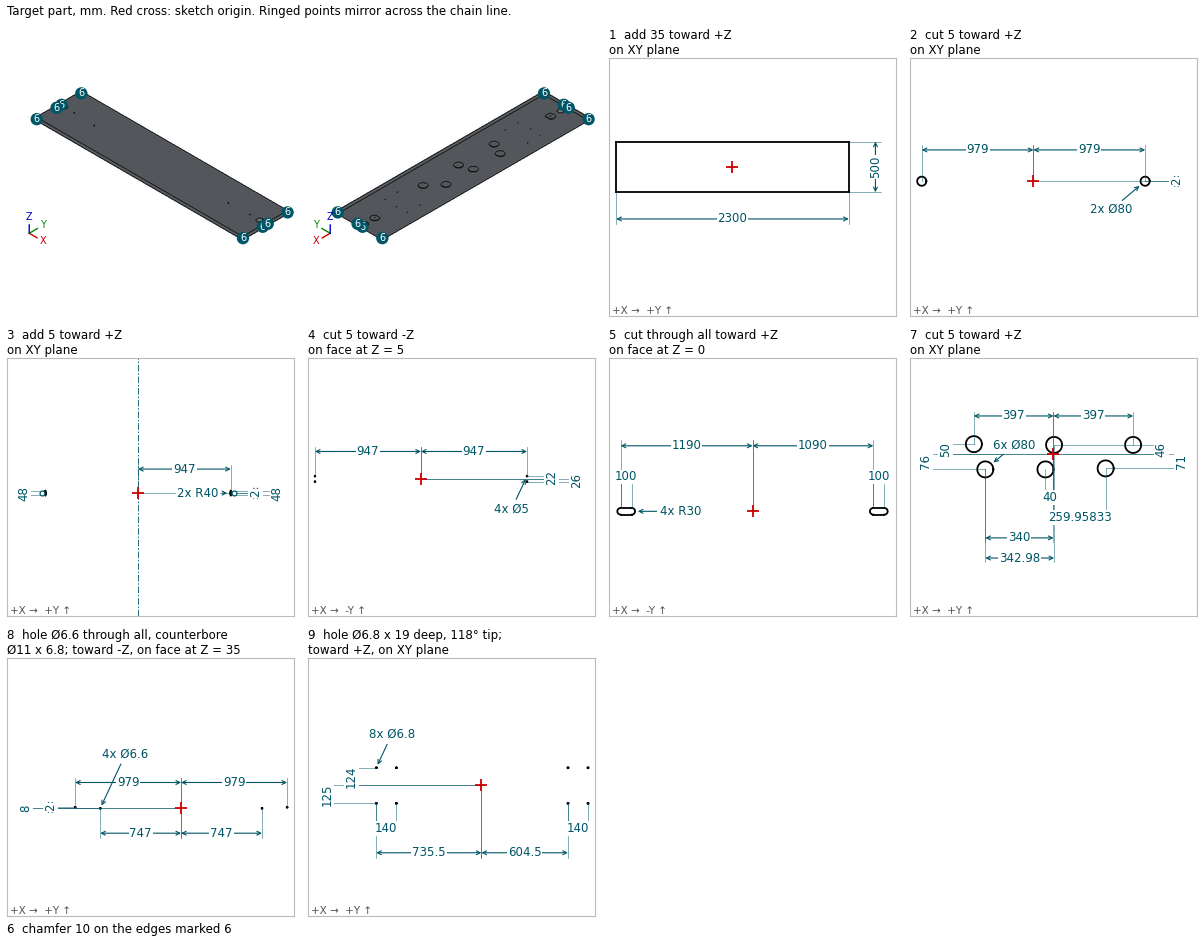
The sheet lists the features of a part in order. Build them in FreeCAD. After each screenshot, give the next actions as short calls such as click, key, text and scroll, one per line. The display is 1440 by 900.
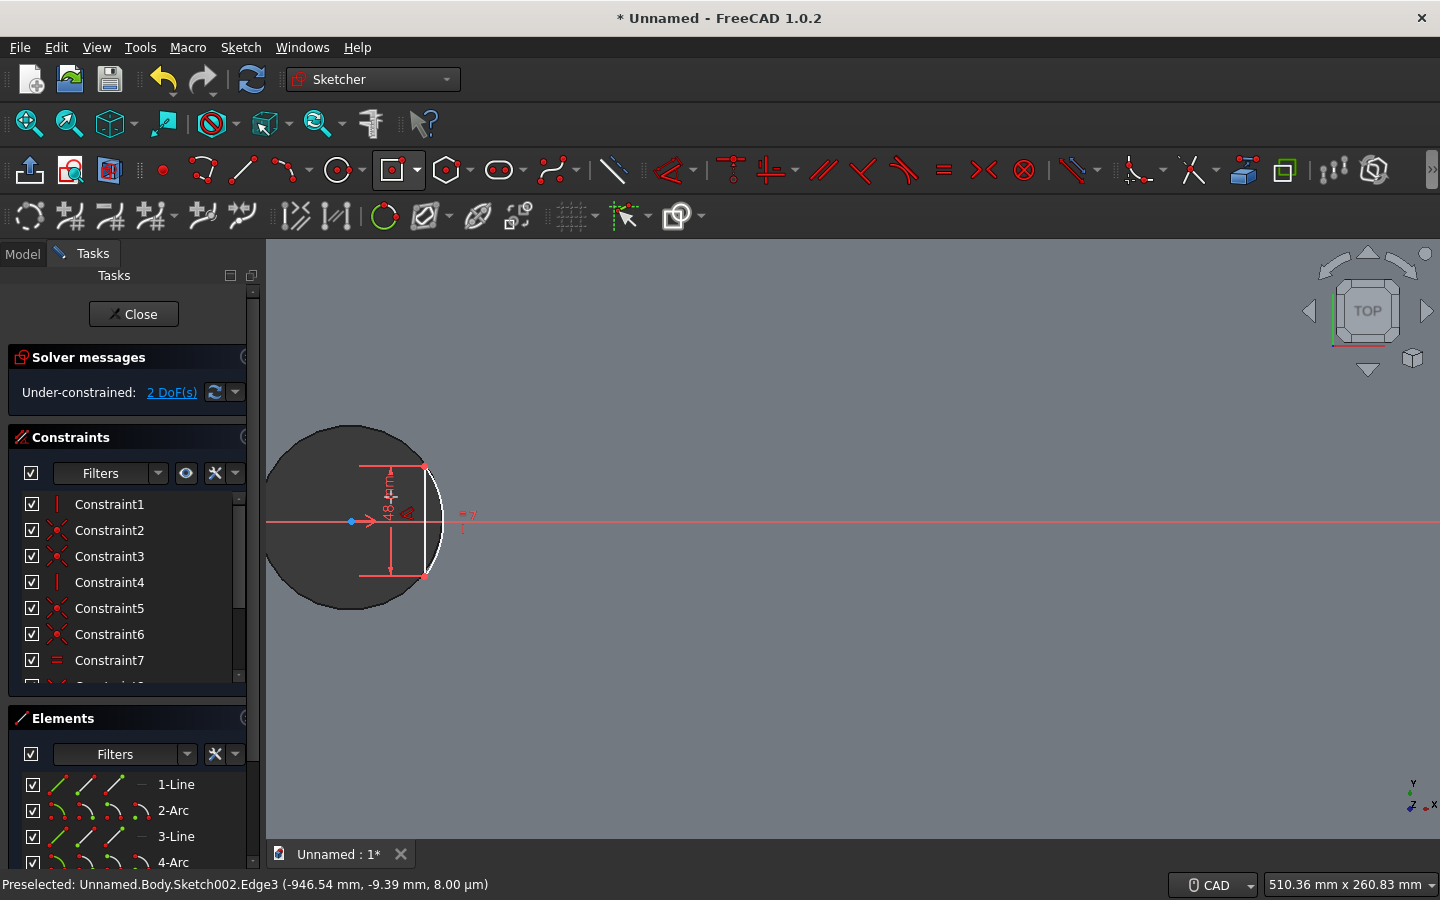
scroll(424, 543, down, 9)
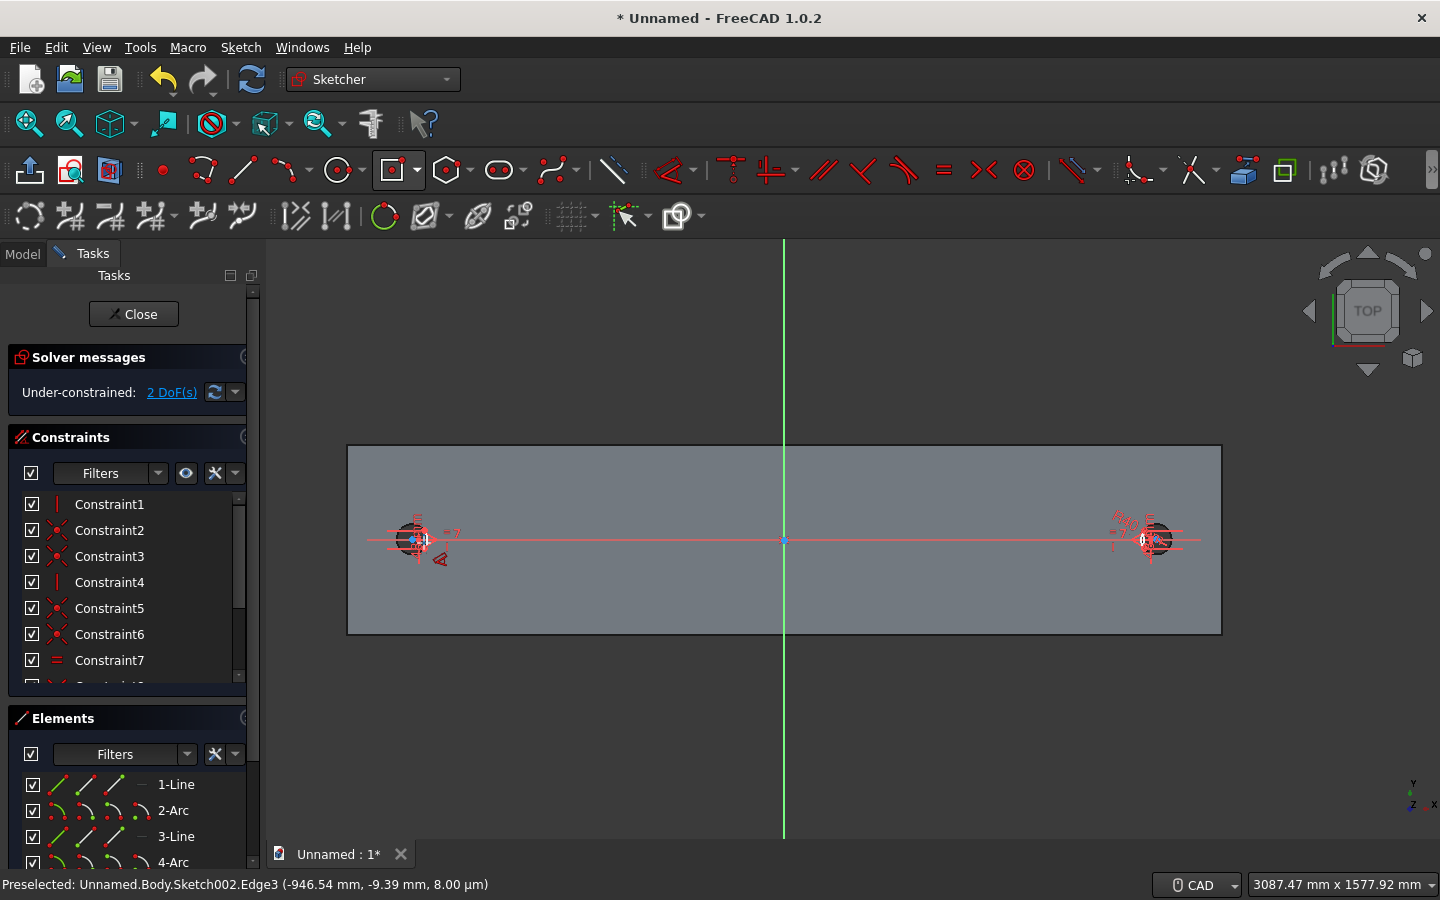
scroll(1156, 540, up, 20)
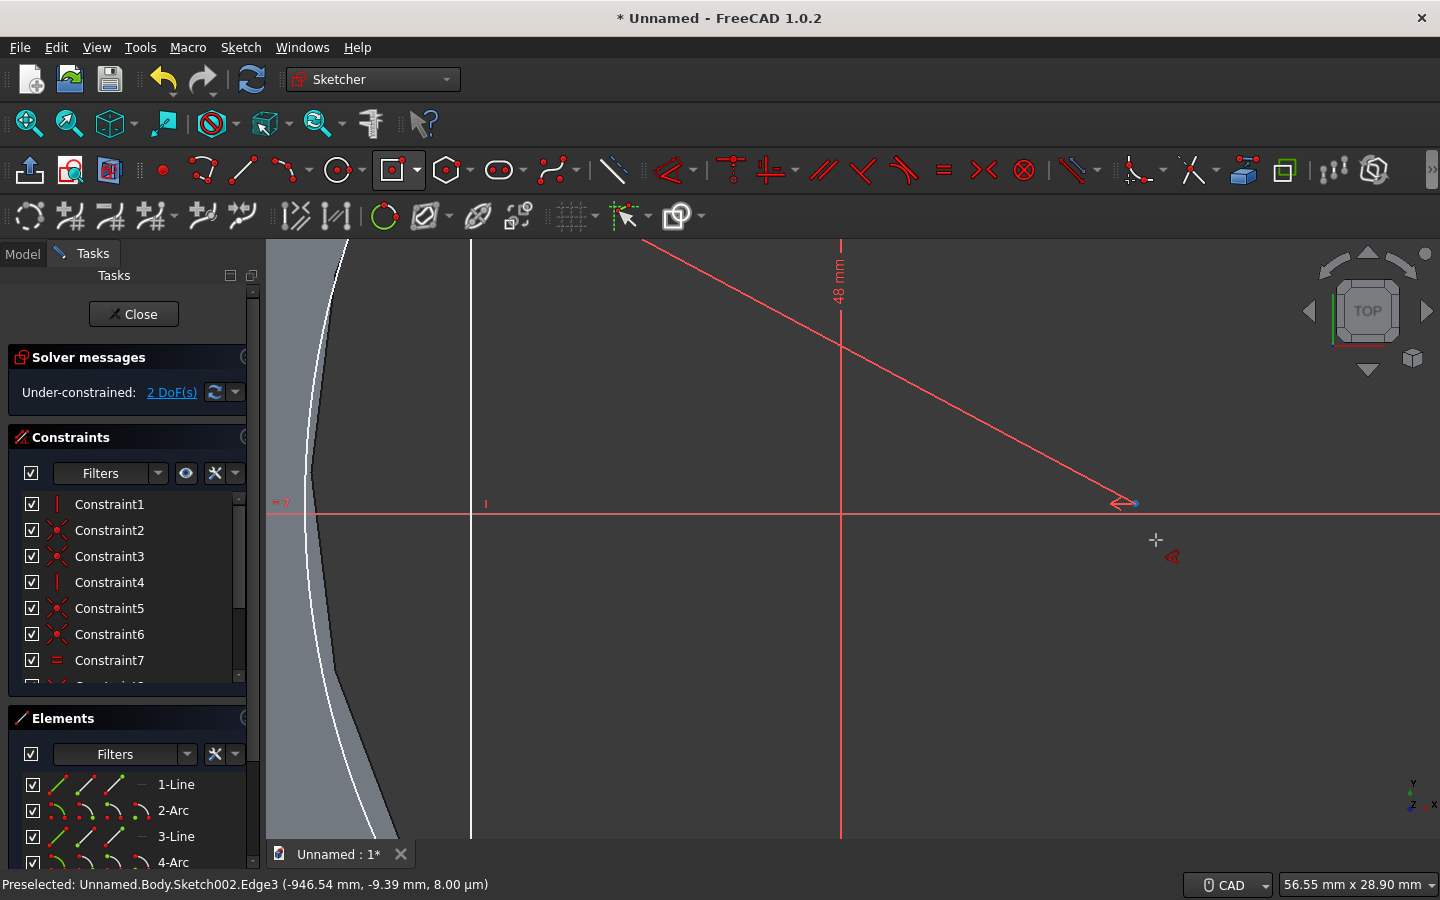
click(1135, 504)
click(1169, 506)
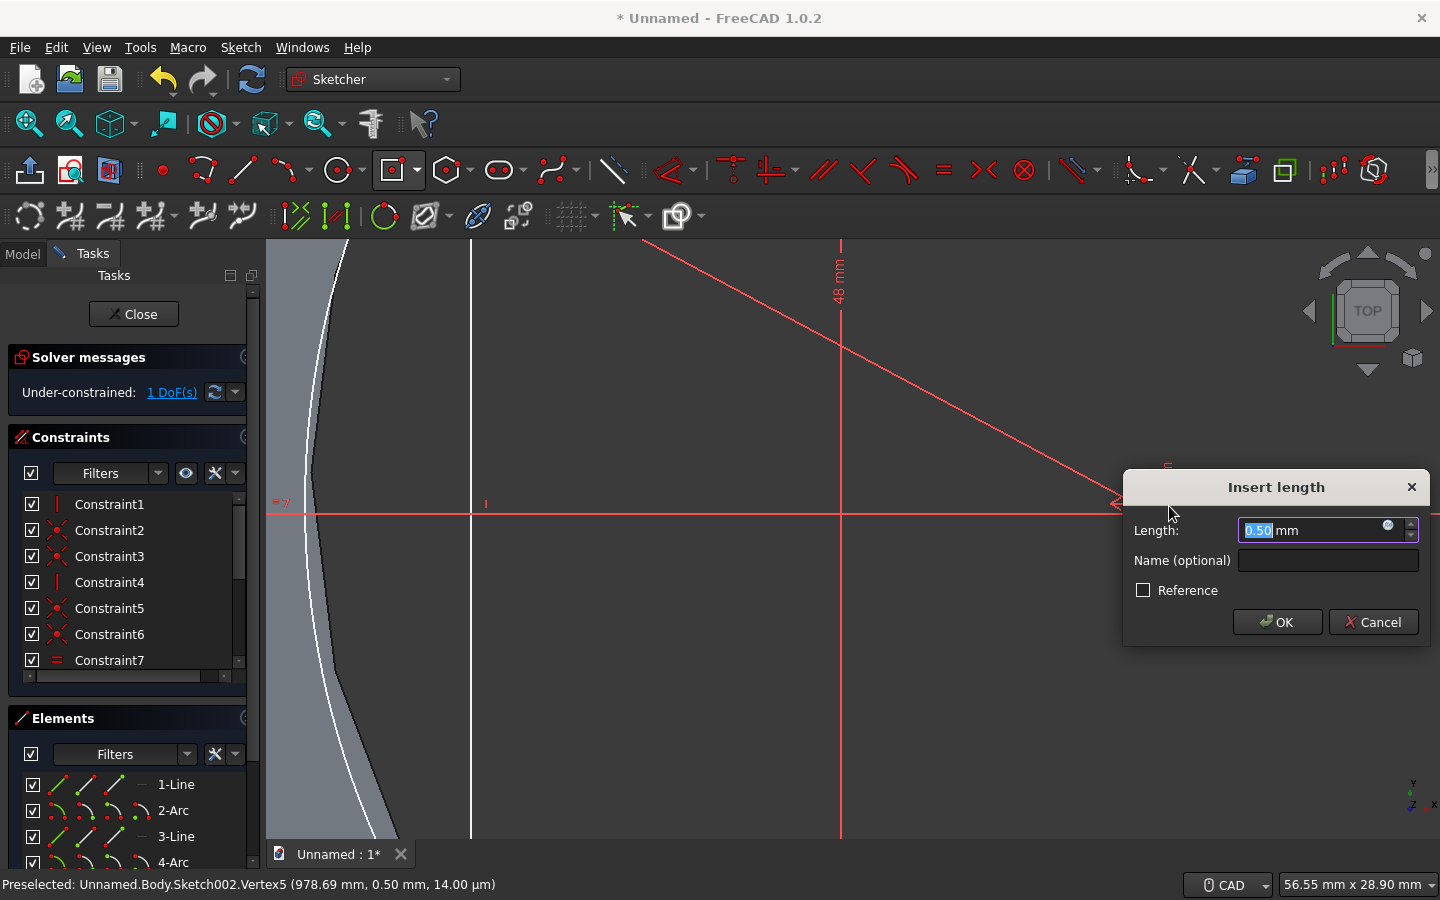
text(2)
key(Return)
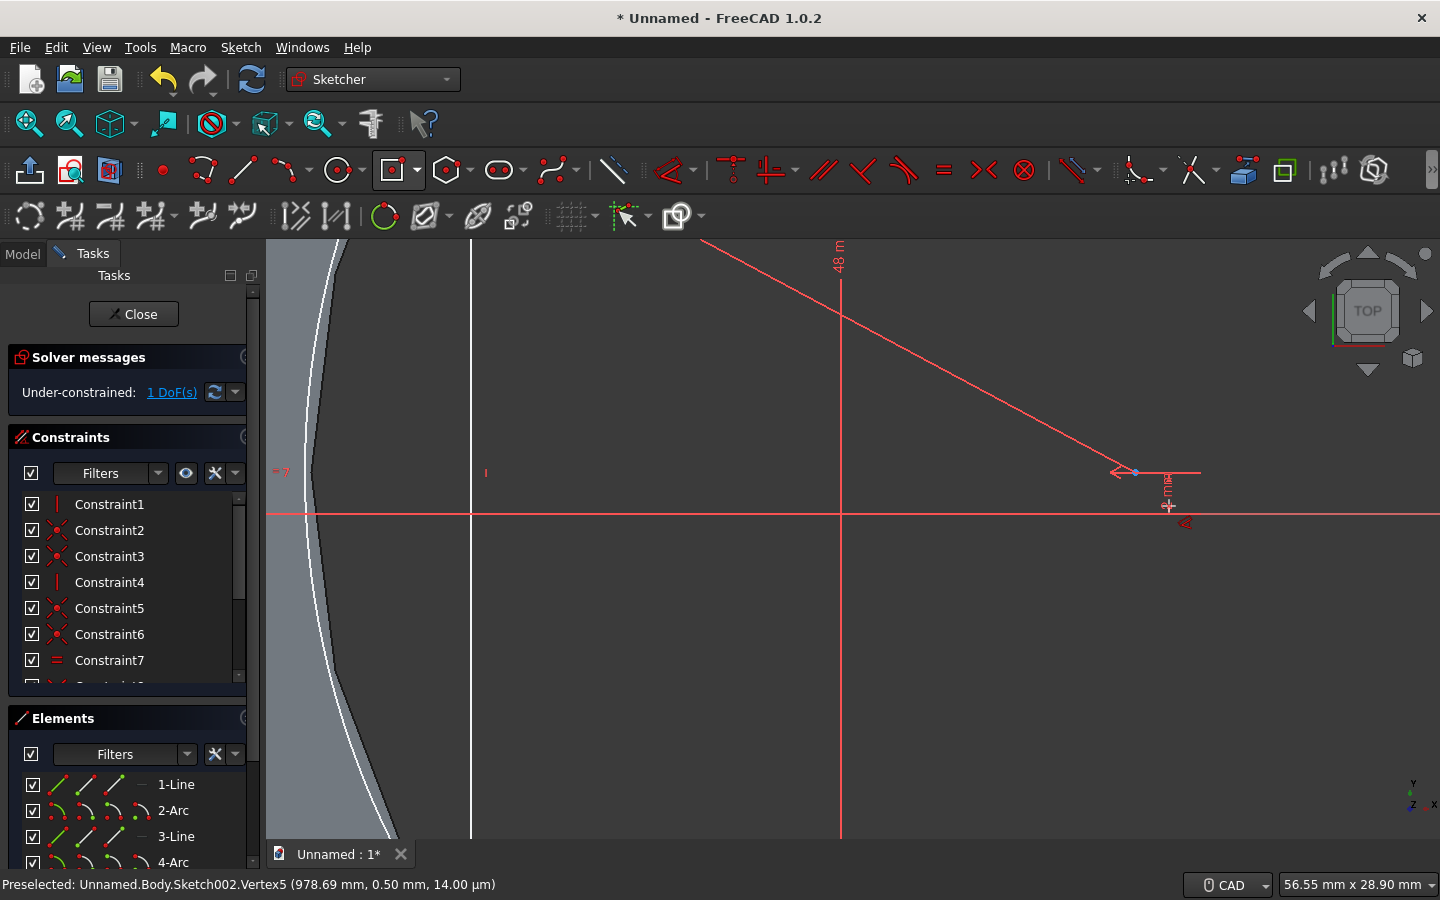
scroll(784, 539, down, 15)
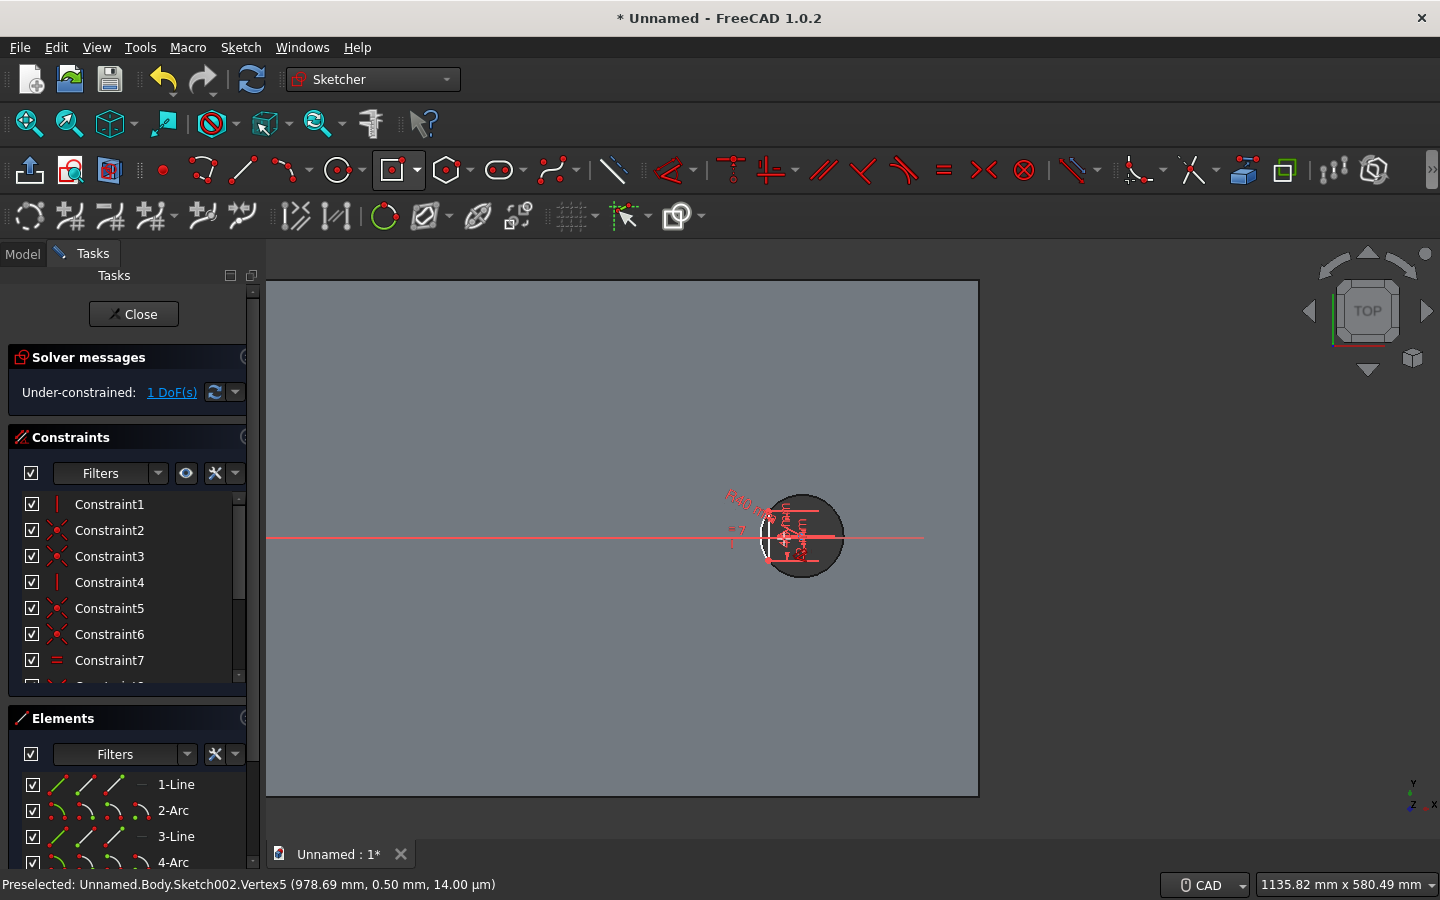
scroll(1275, 541, down, 5)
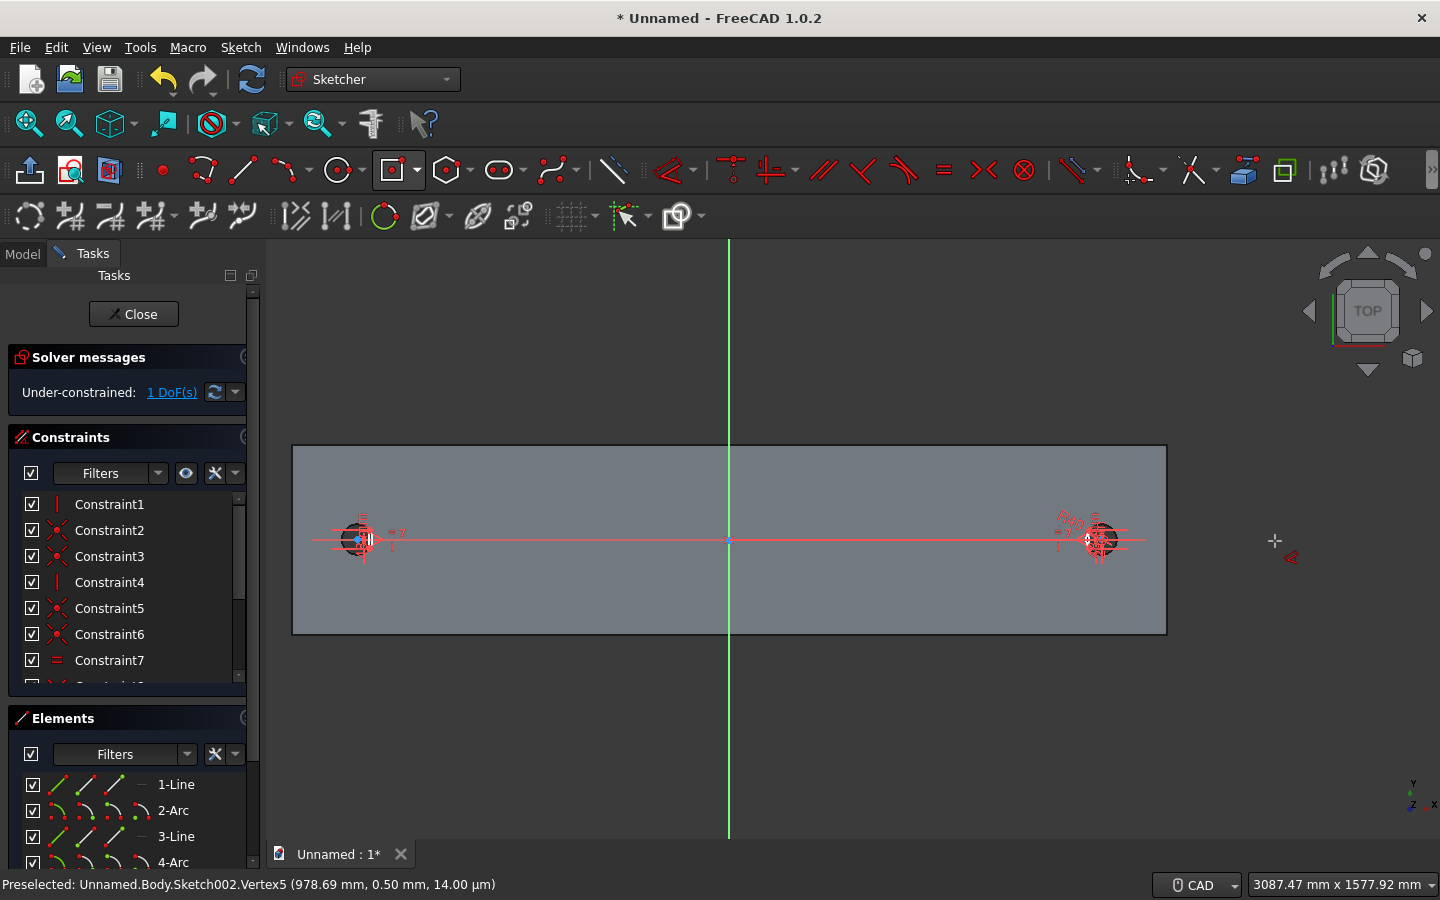
click(1089, 530)
click(909, 496)